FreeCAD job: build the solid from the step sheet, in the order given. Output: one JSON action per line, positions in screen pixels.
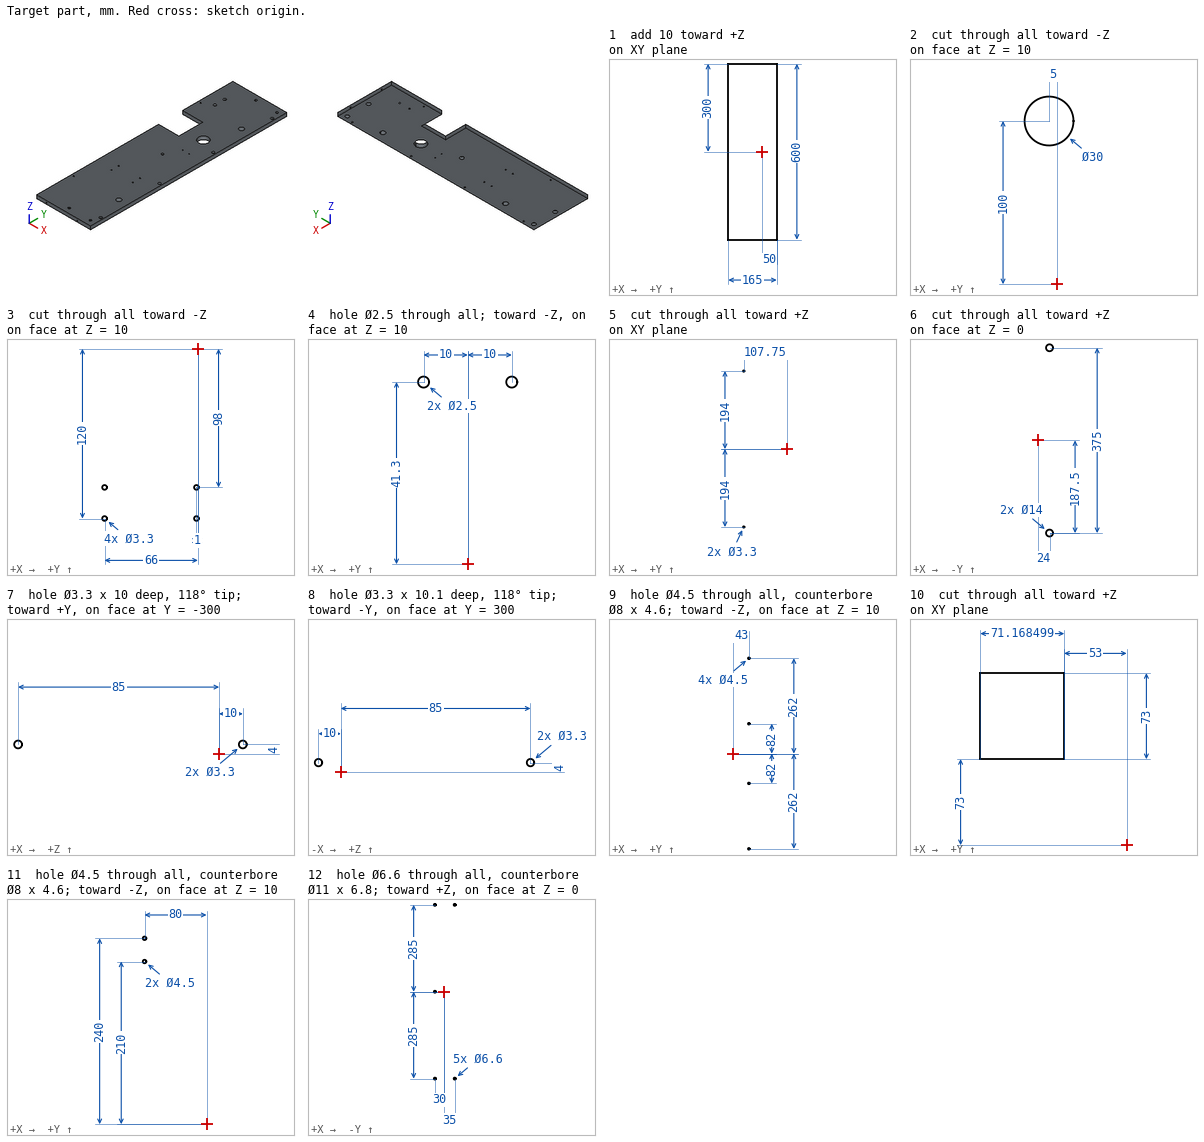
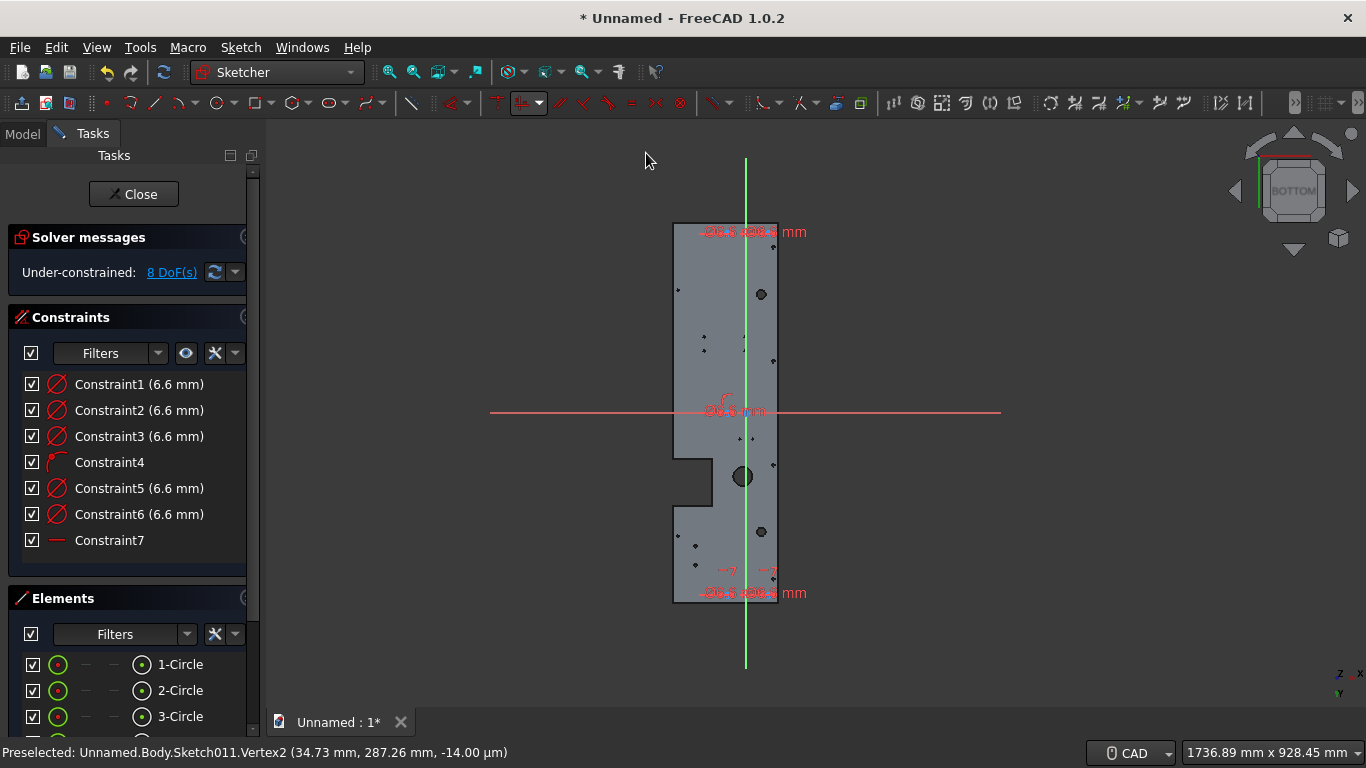
{"action": "left_click", "coordinate": [727, 595]}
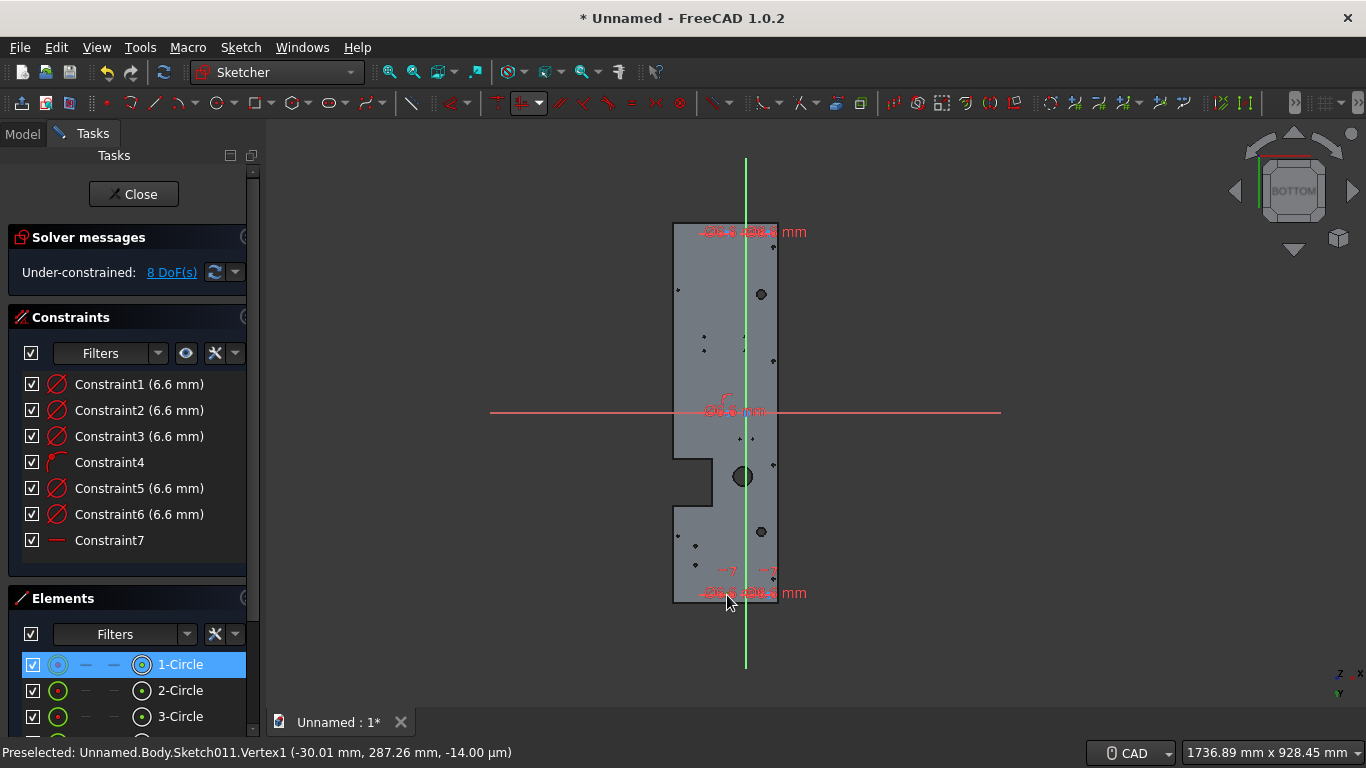
{"action": "left_click", "coordinate": [727, 413]}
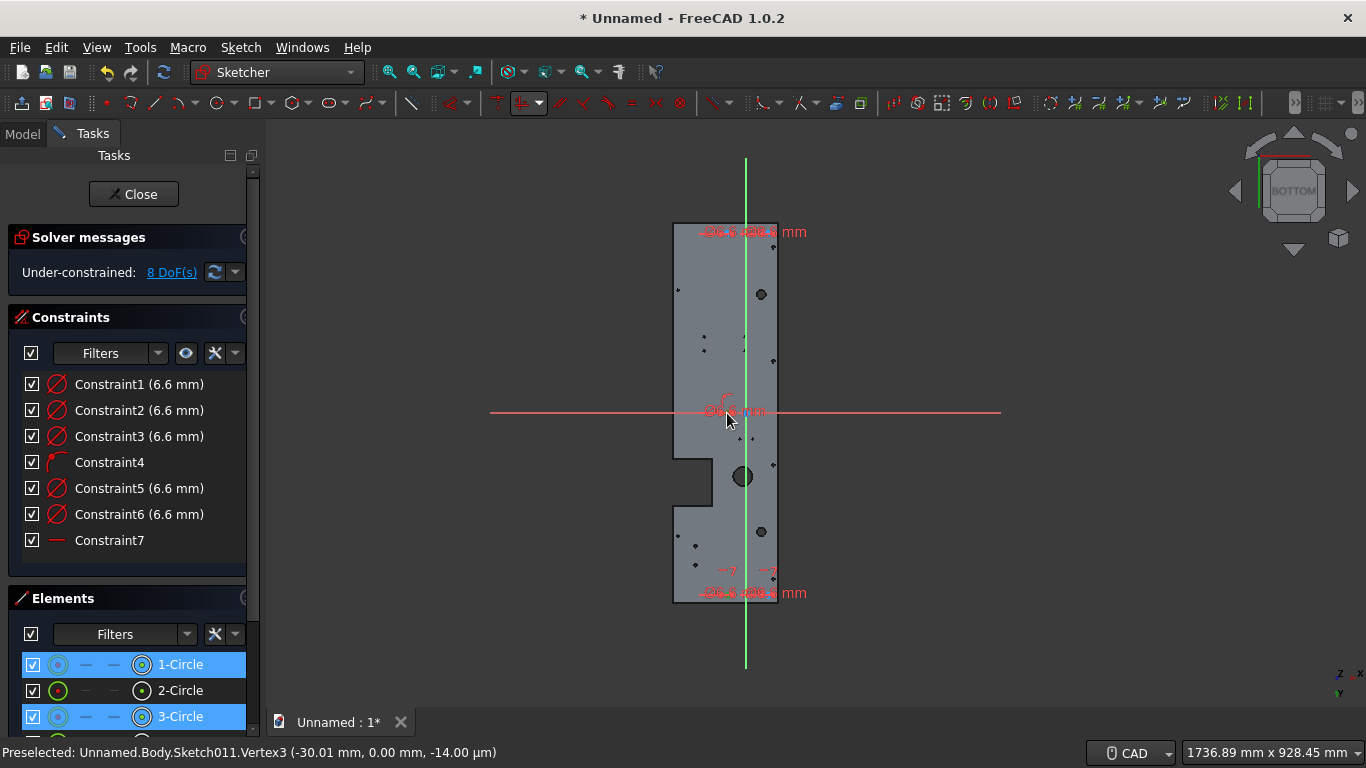
{"action": "left_click", "coordinate": [542, 104]}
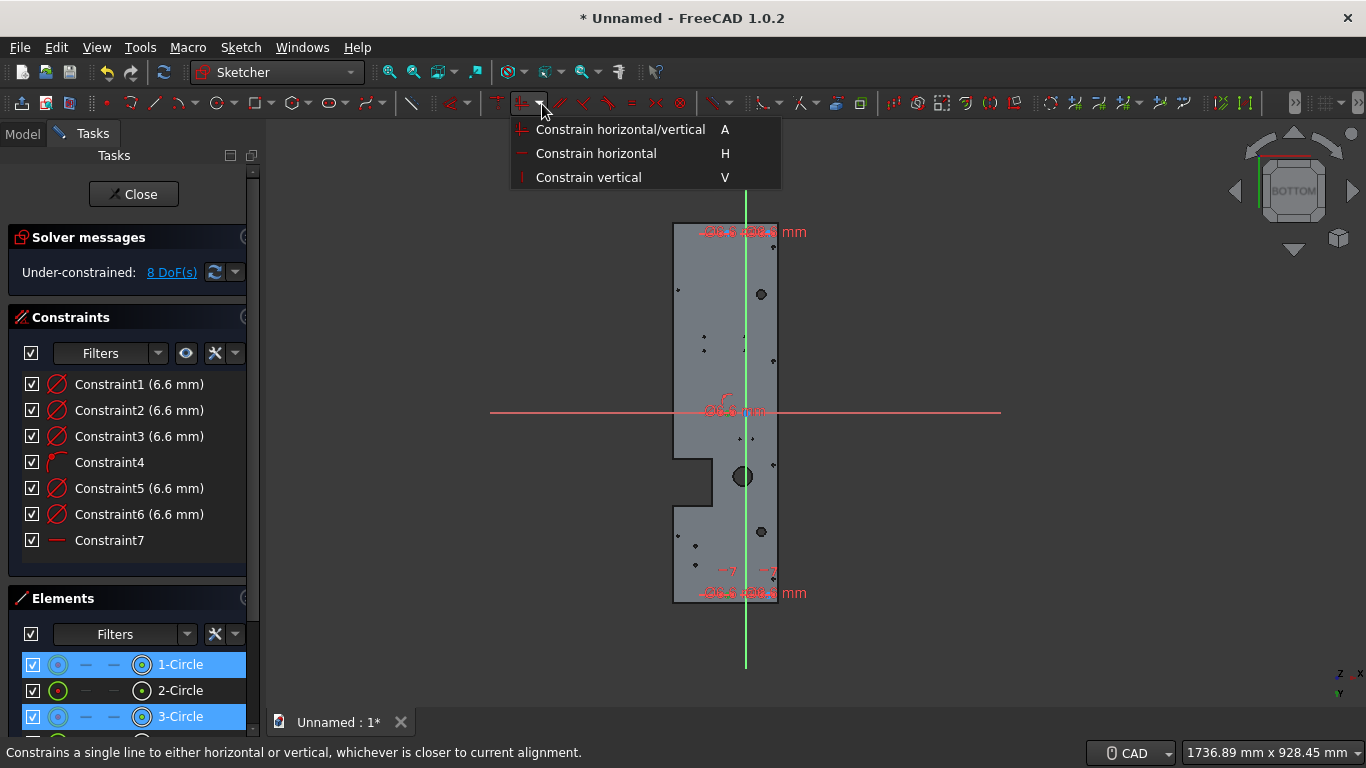
{"action": "left_click", "coordinate": [646, 177]}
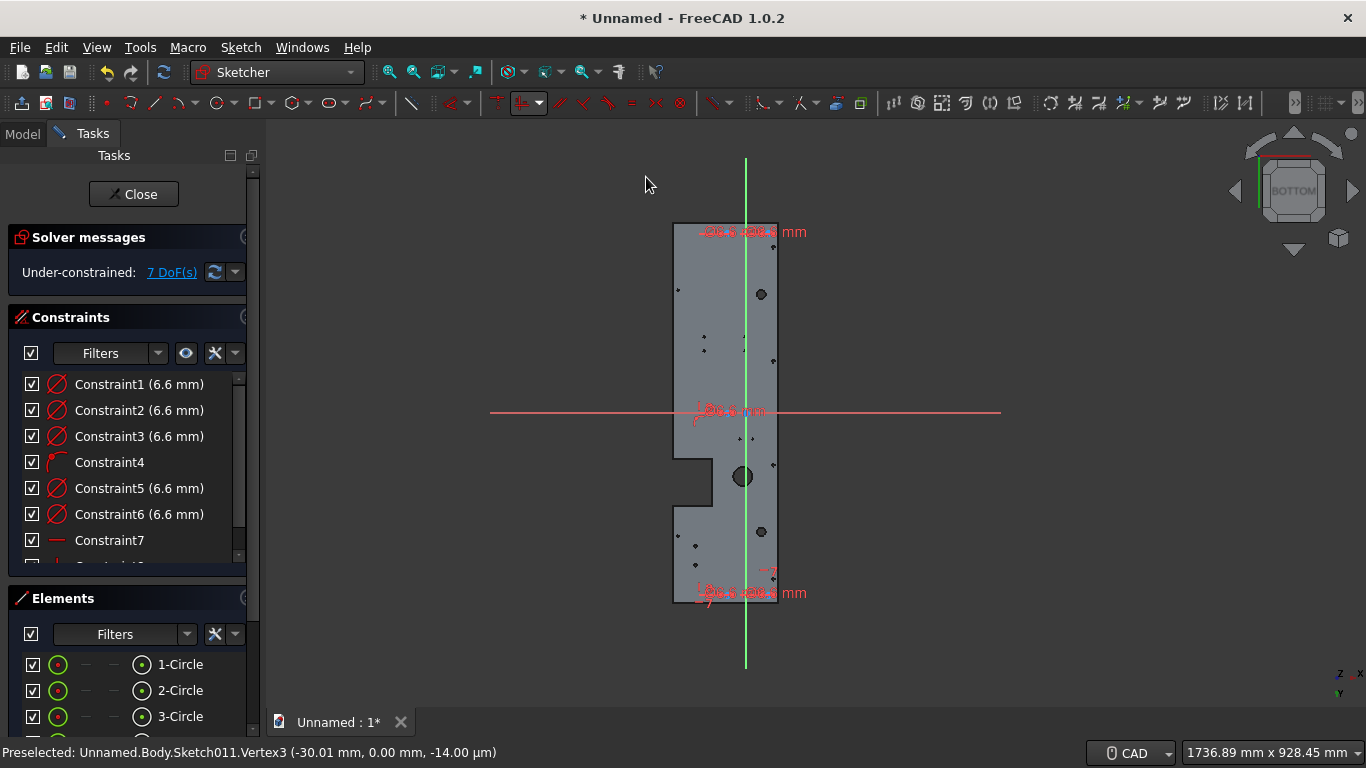
{"action": "left_click", "coordinate": [727, 413]}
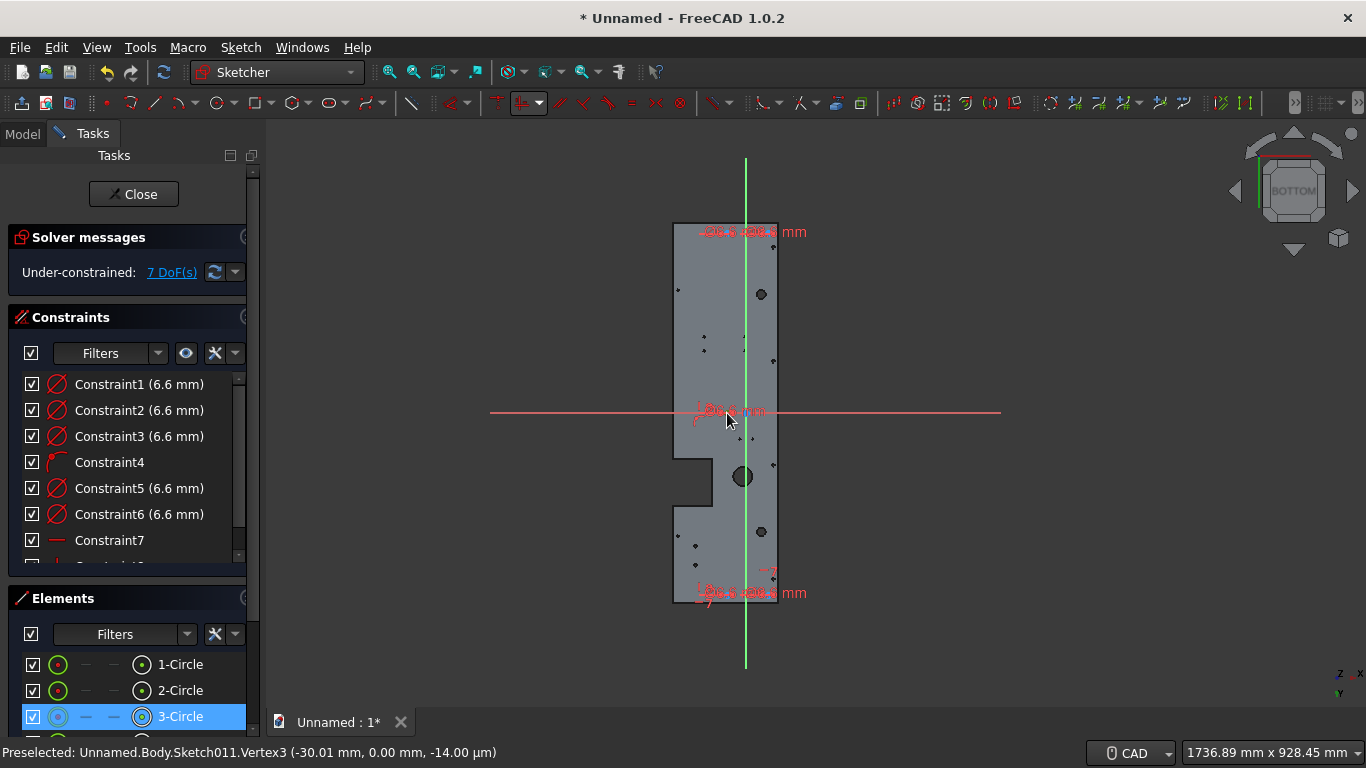
{"action": "left_click", "coordinate": [727, 234]}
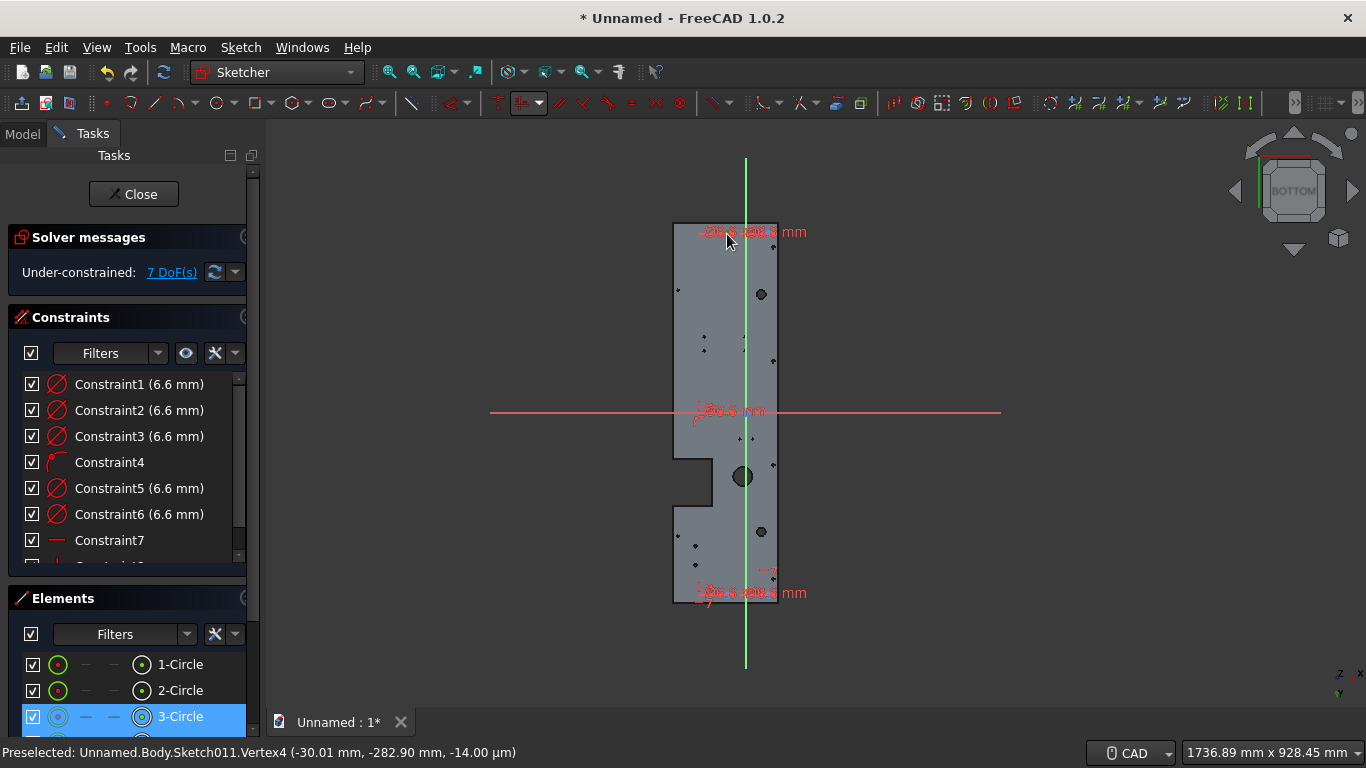
{"action": "key", "text": "v"}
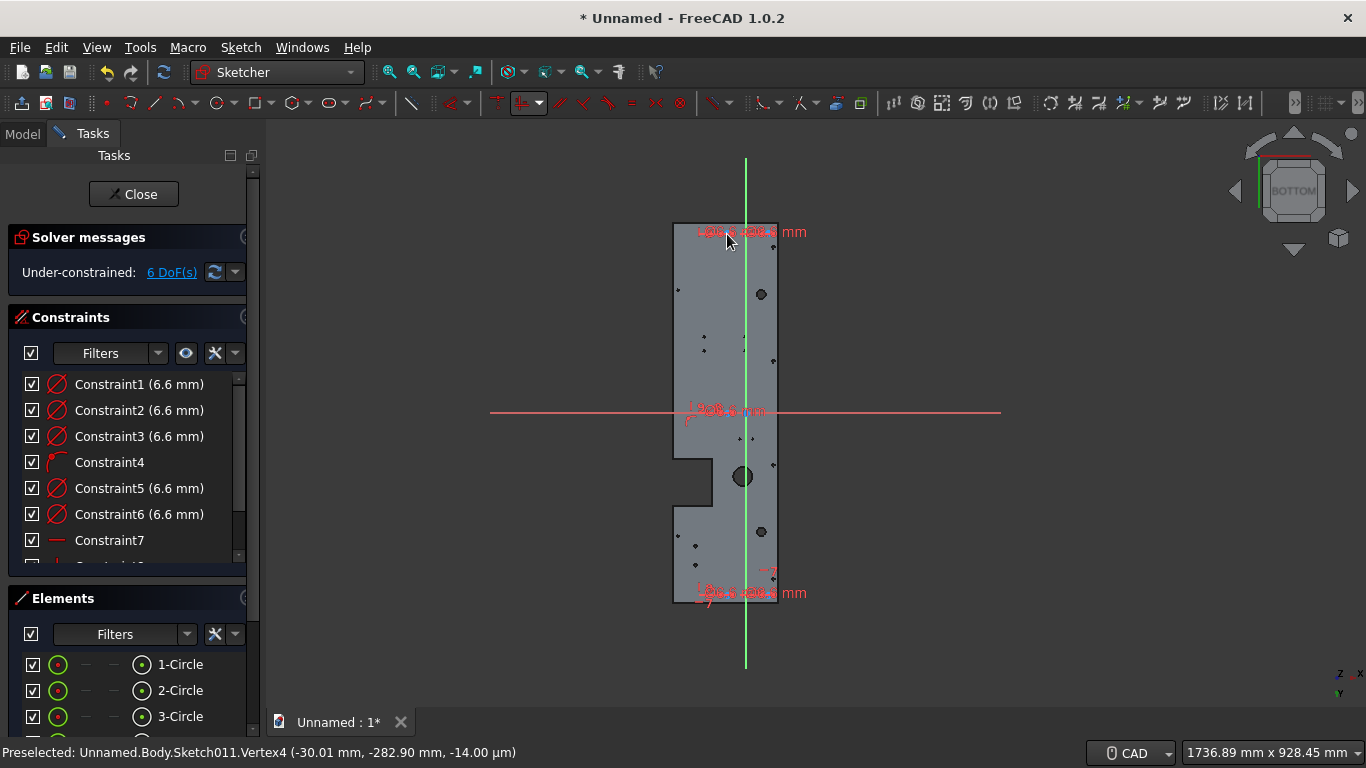
{"action": "left_click", "coordinate": [768, 595]}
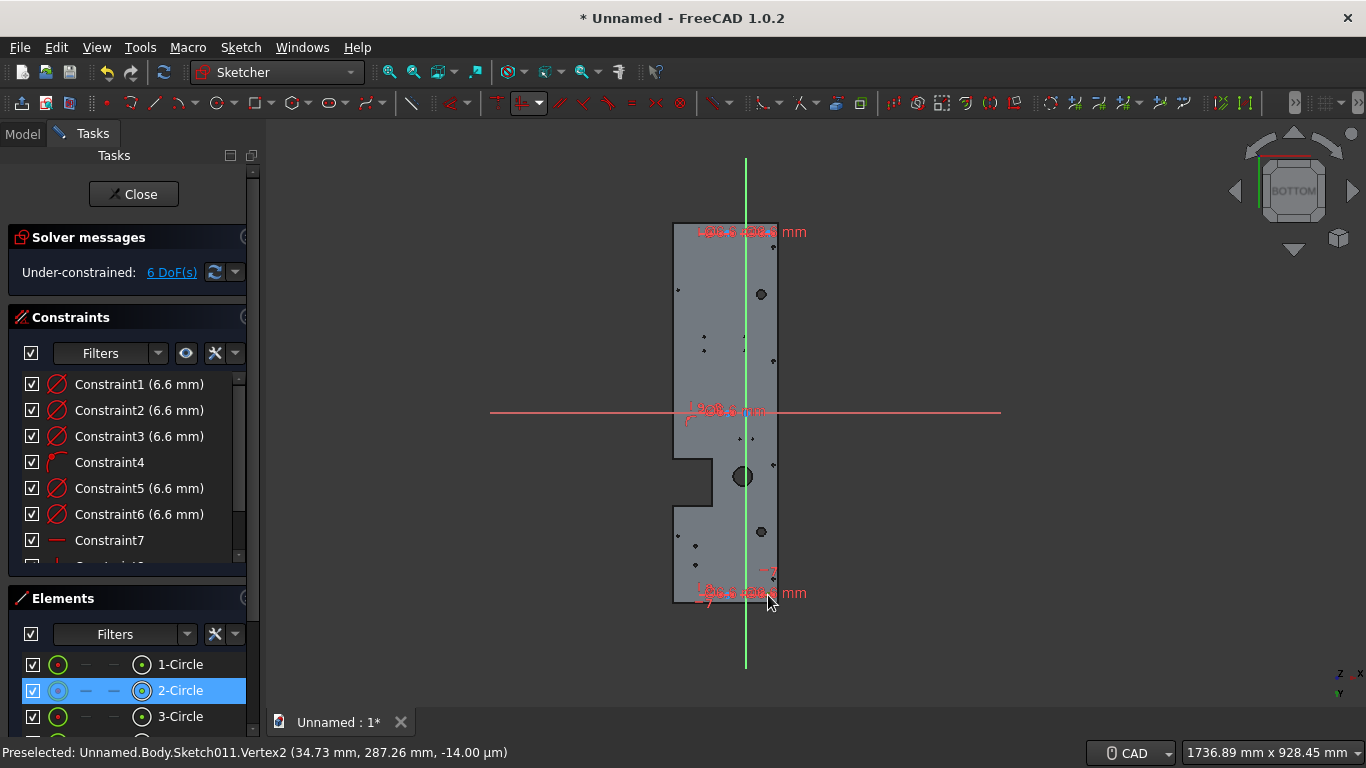
{"action": "left_click", "coordinate": [768, 234]}